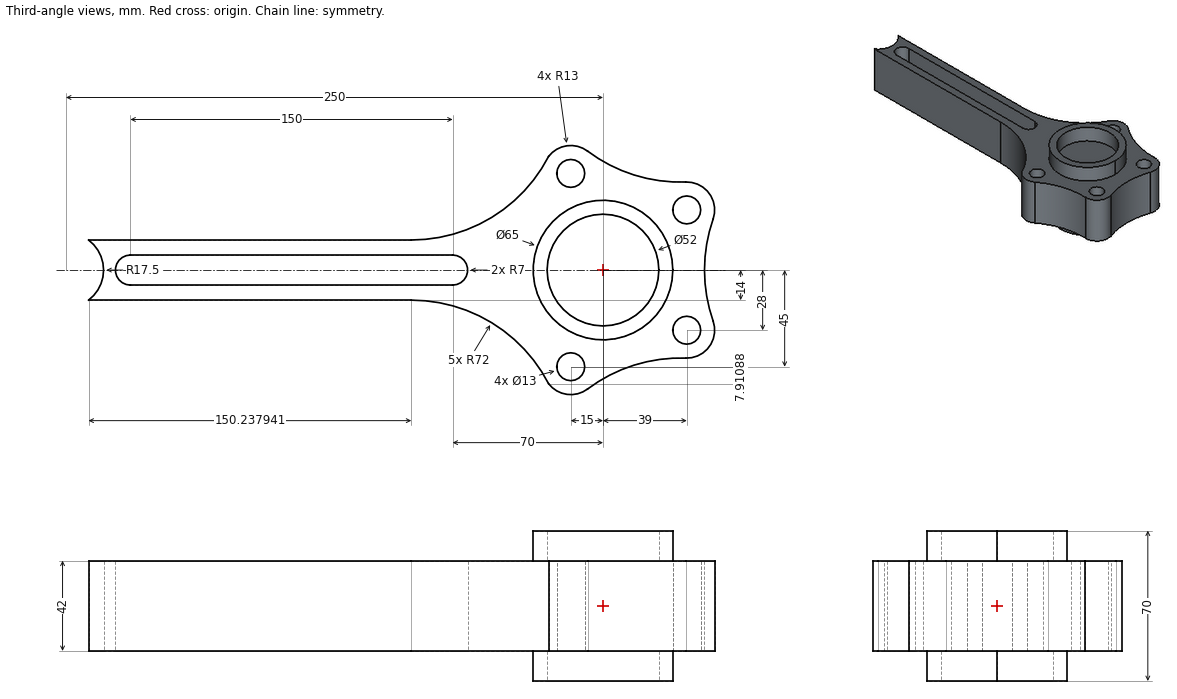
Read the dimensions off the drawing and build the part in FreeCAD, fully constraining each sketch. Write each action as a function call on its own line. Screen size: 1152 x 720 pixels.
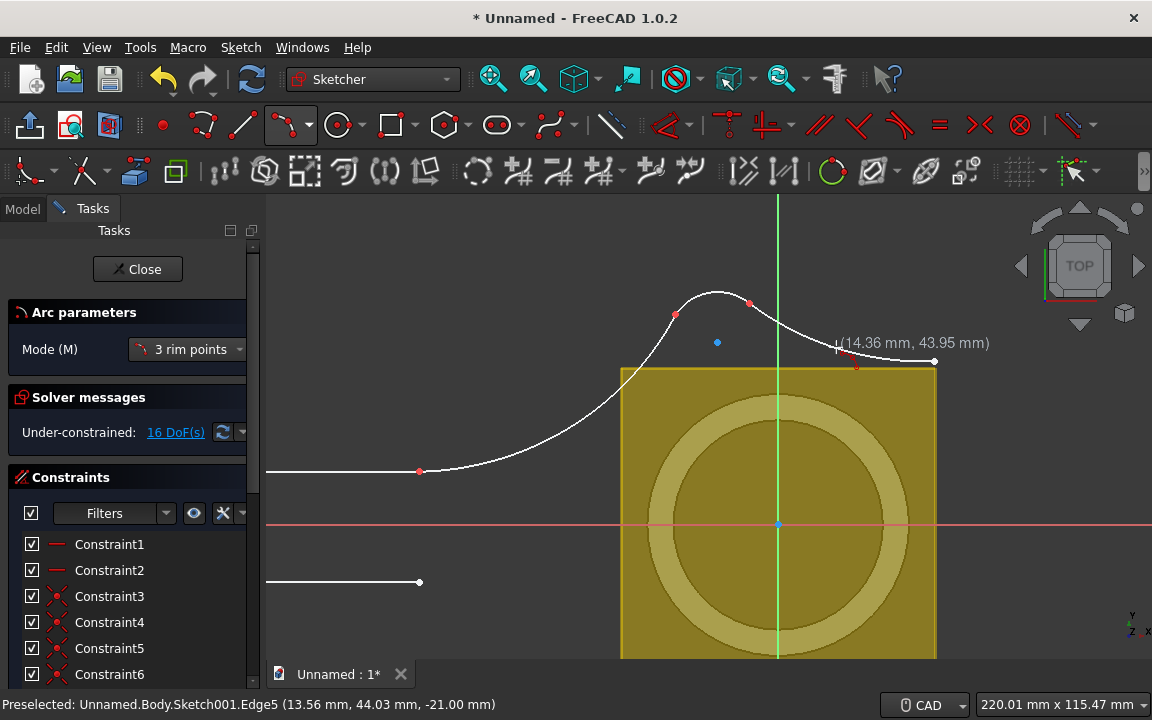
click(934, 361)
click(985, 429)
click(977, 381)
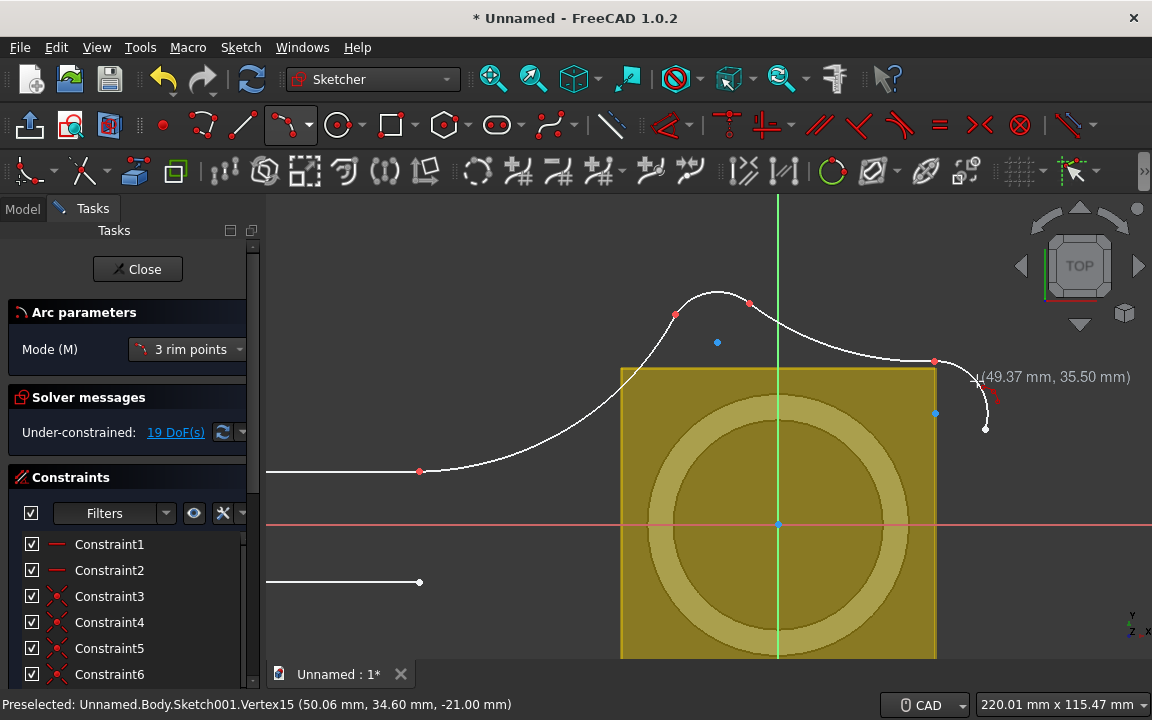
click(985, 430)
click(985, 620)
click(969, 506)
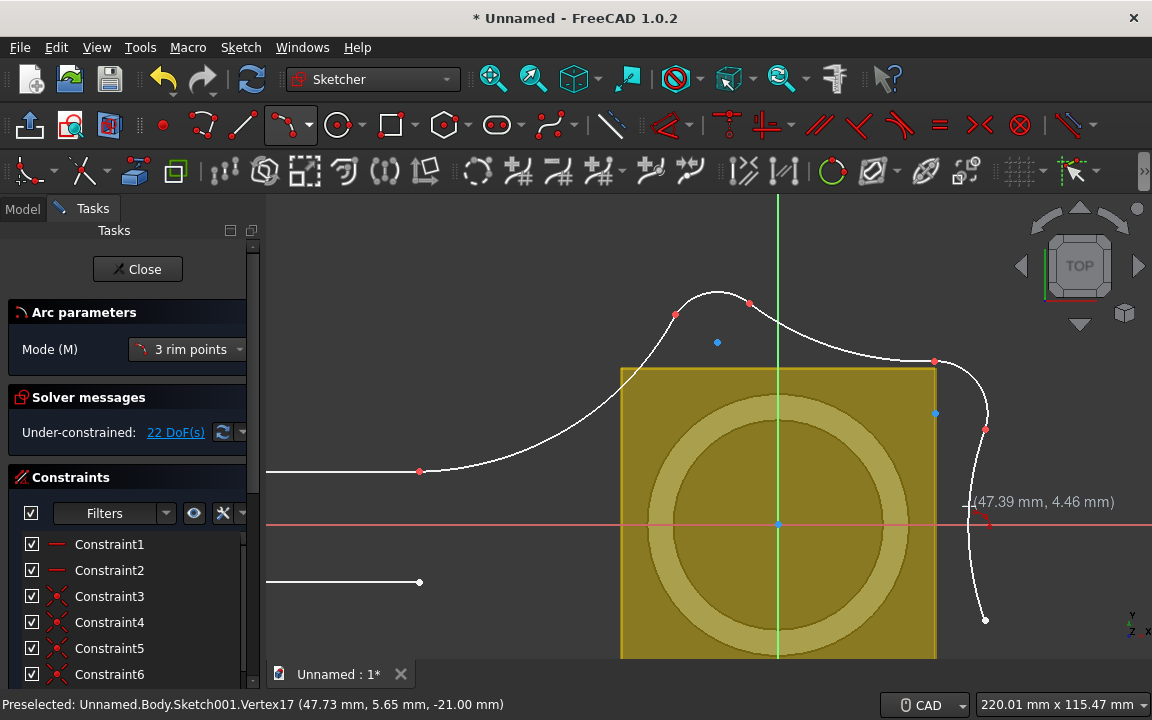
click(985, 621)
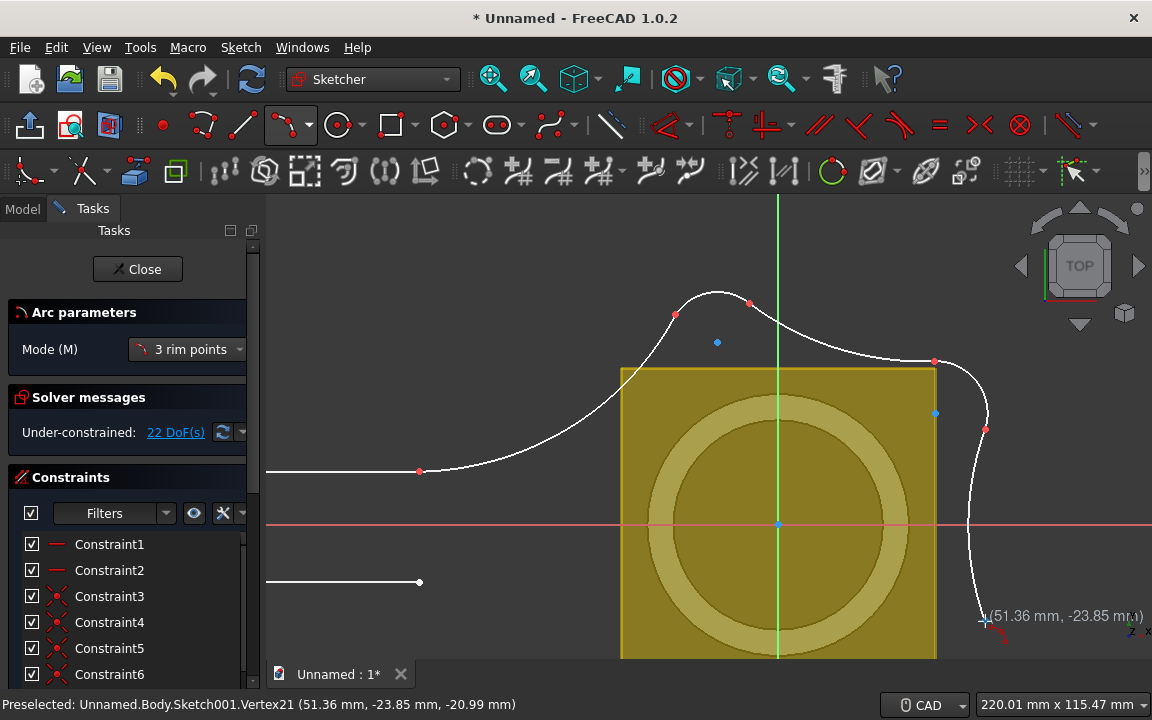
scroll(837, 346, down, 4)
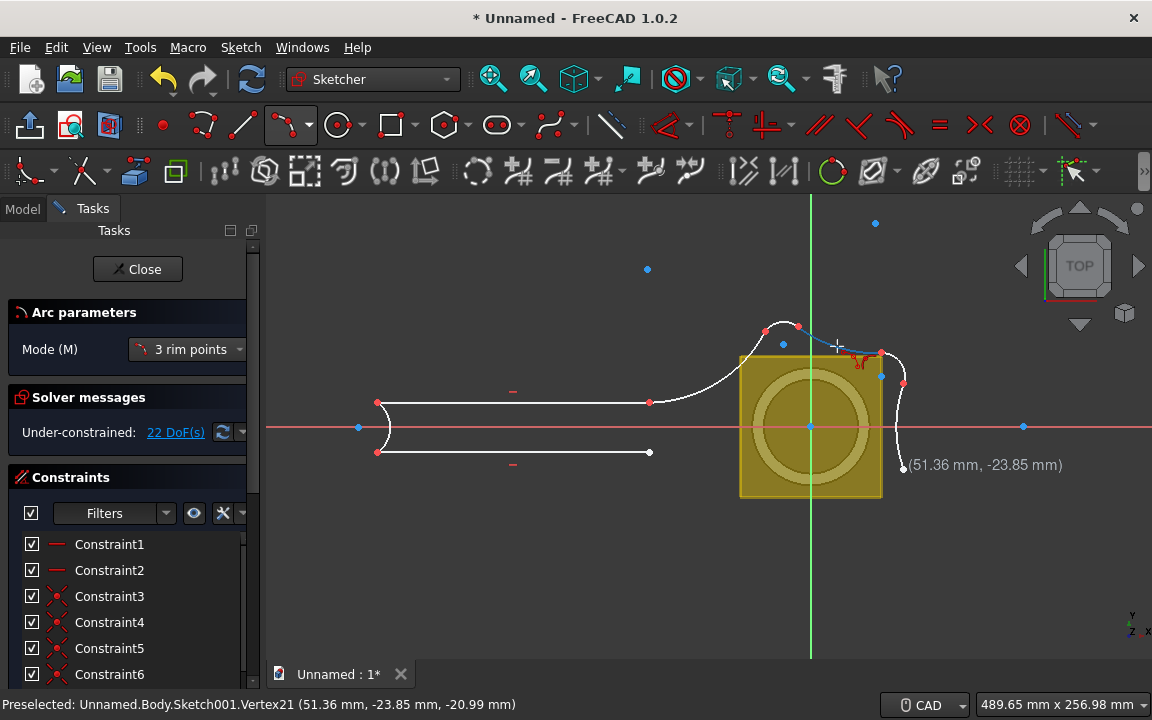
click(881, 501)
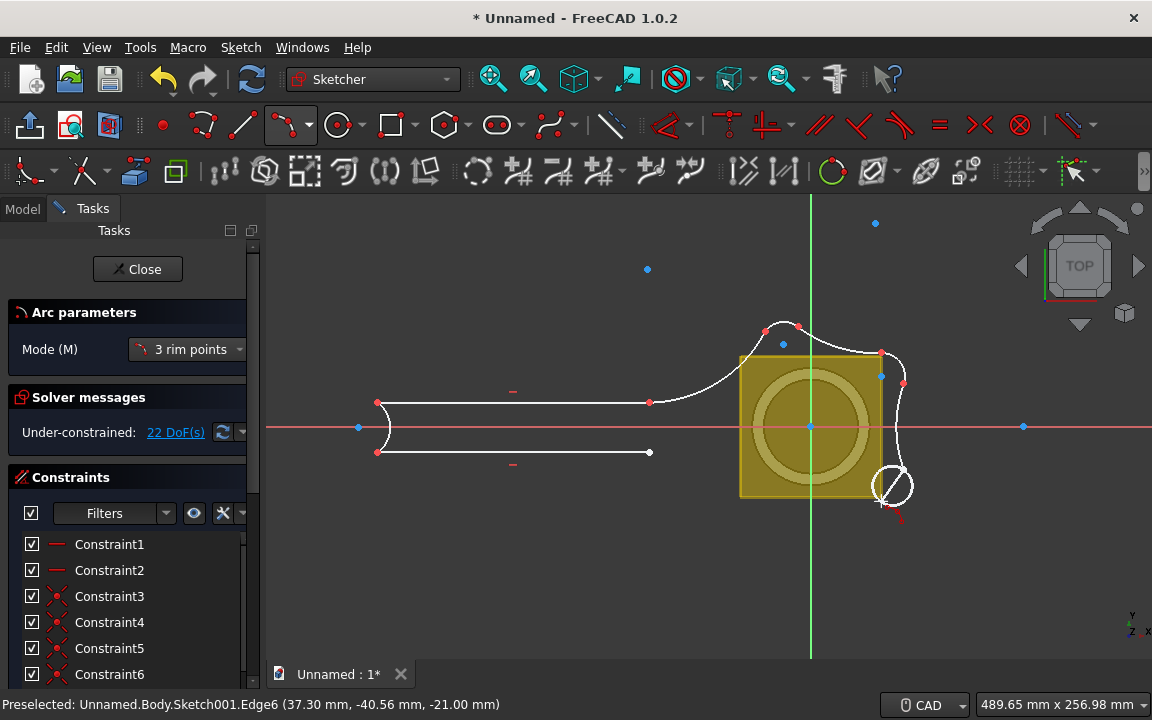
scroll(900, 491, up, 3)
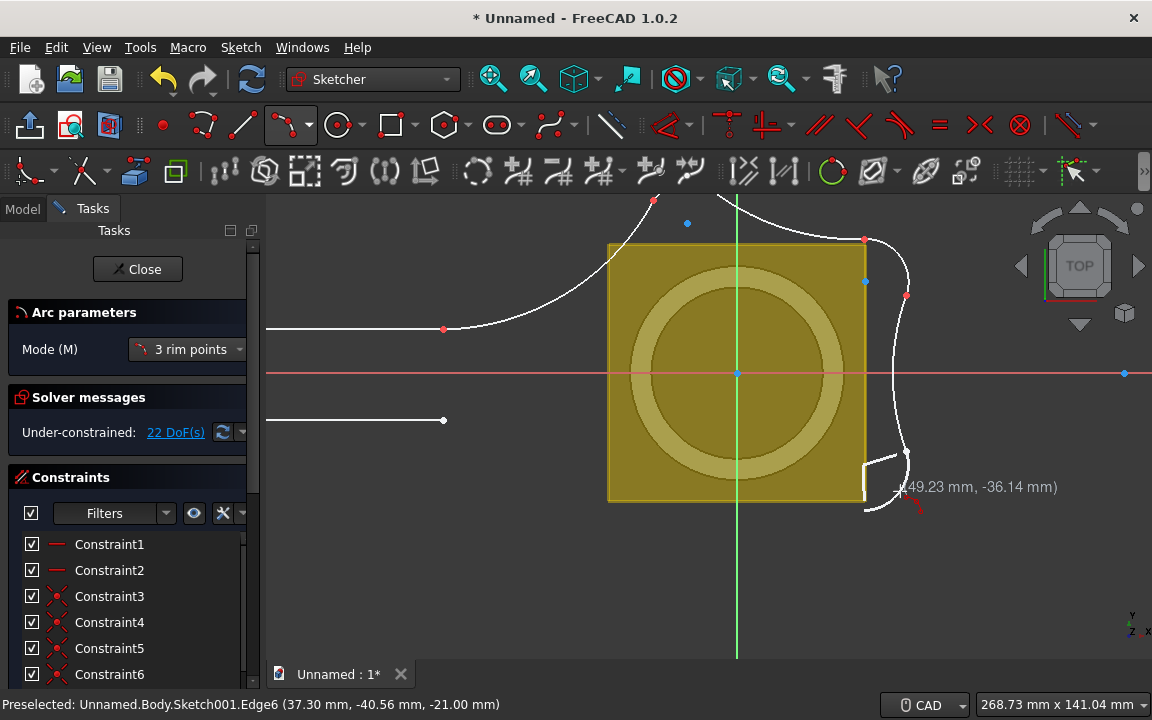
click(900, 491)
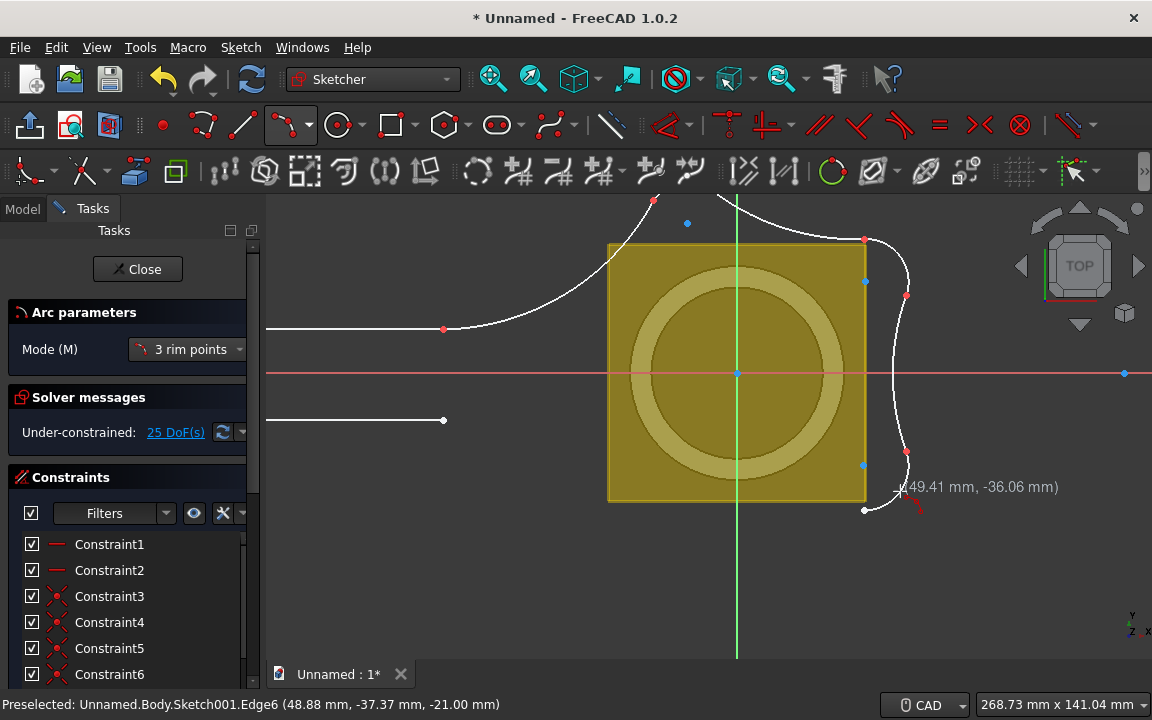
click(865, 511)
click(713, 556)
click(785, 519)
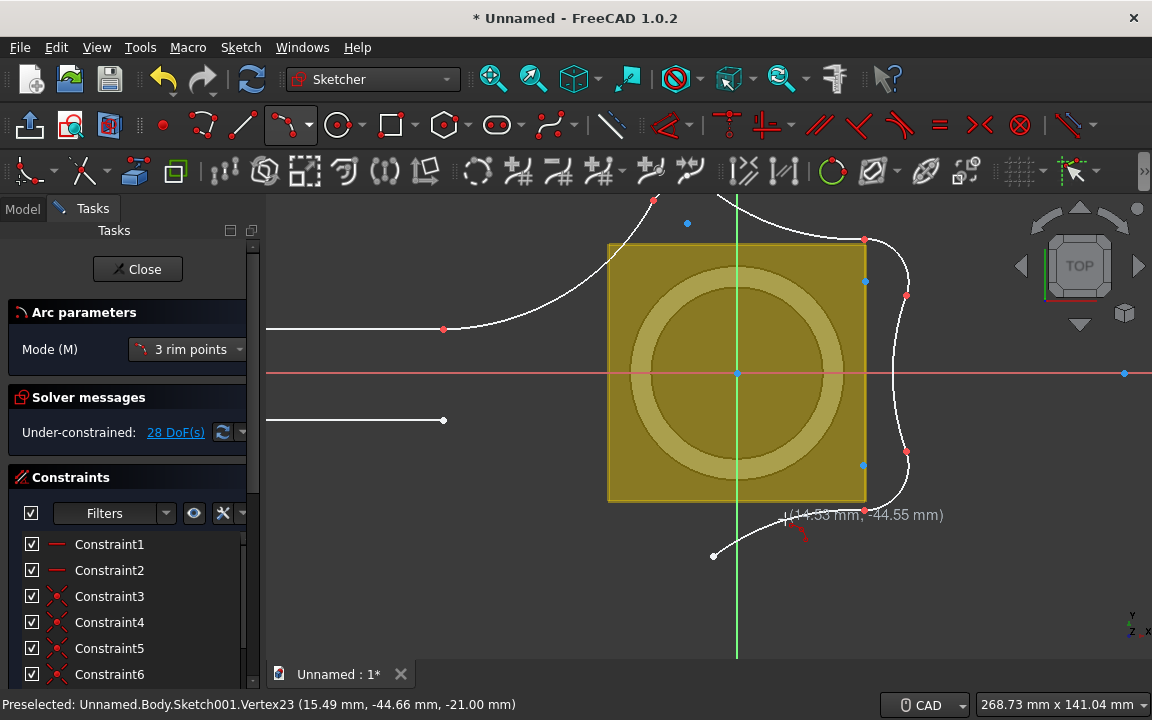
click(713, 557)
click(654, 548)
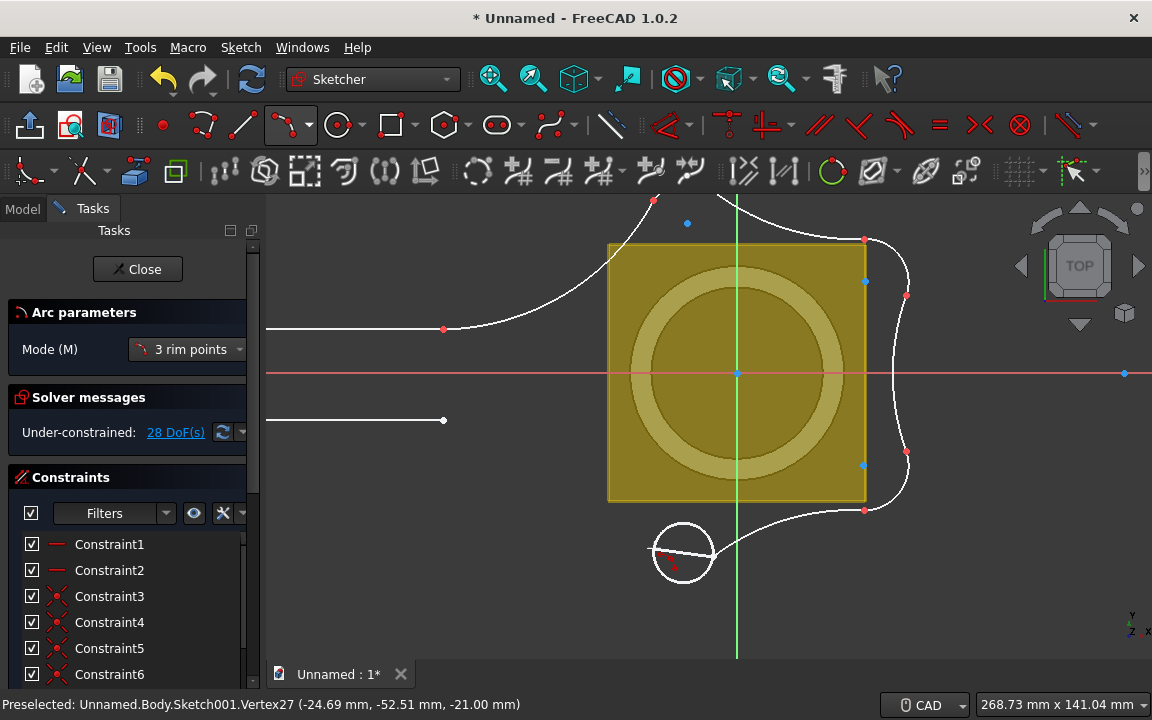
scroll(682, 564, up, 2)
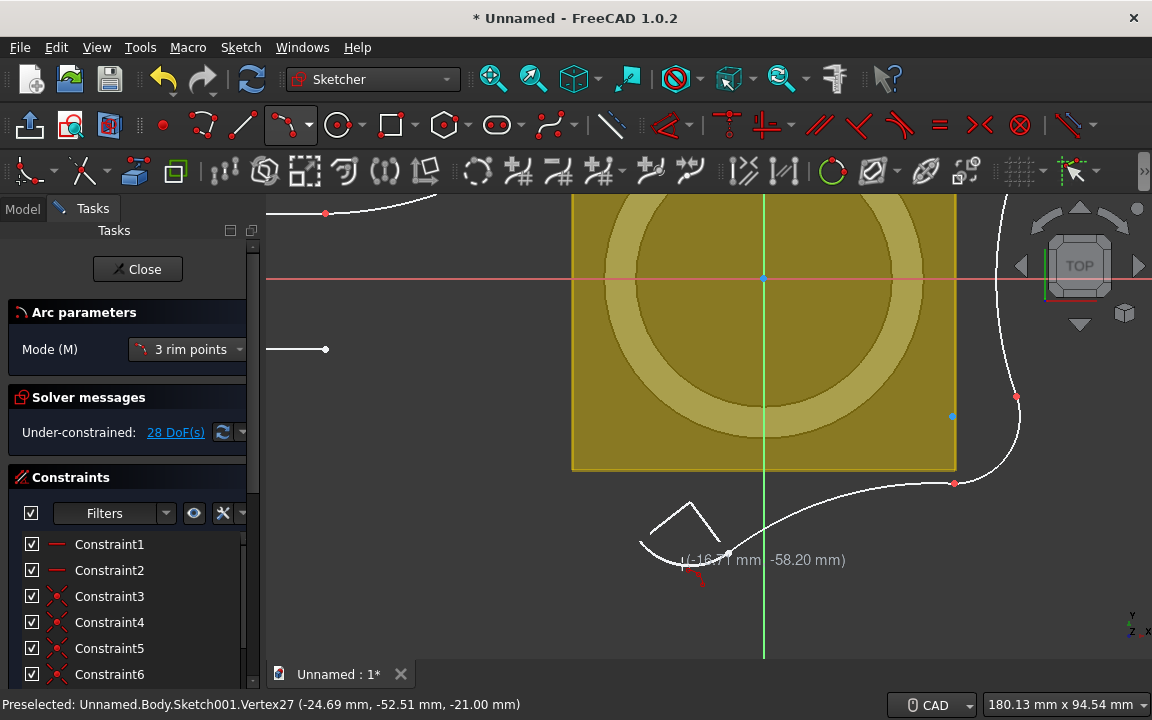
click(682, 564)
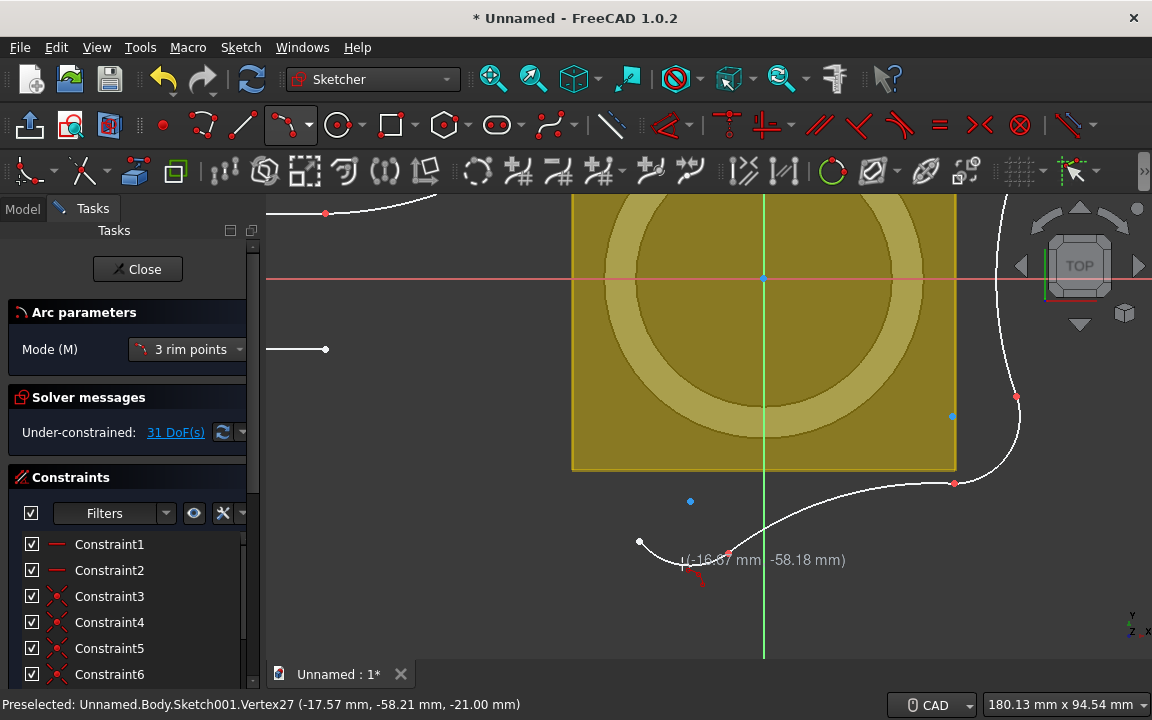
click(640, 541)
click(326, 349)
click(509, 399)